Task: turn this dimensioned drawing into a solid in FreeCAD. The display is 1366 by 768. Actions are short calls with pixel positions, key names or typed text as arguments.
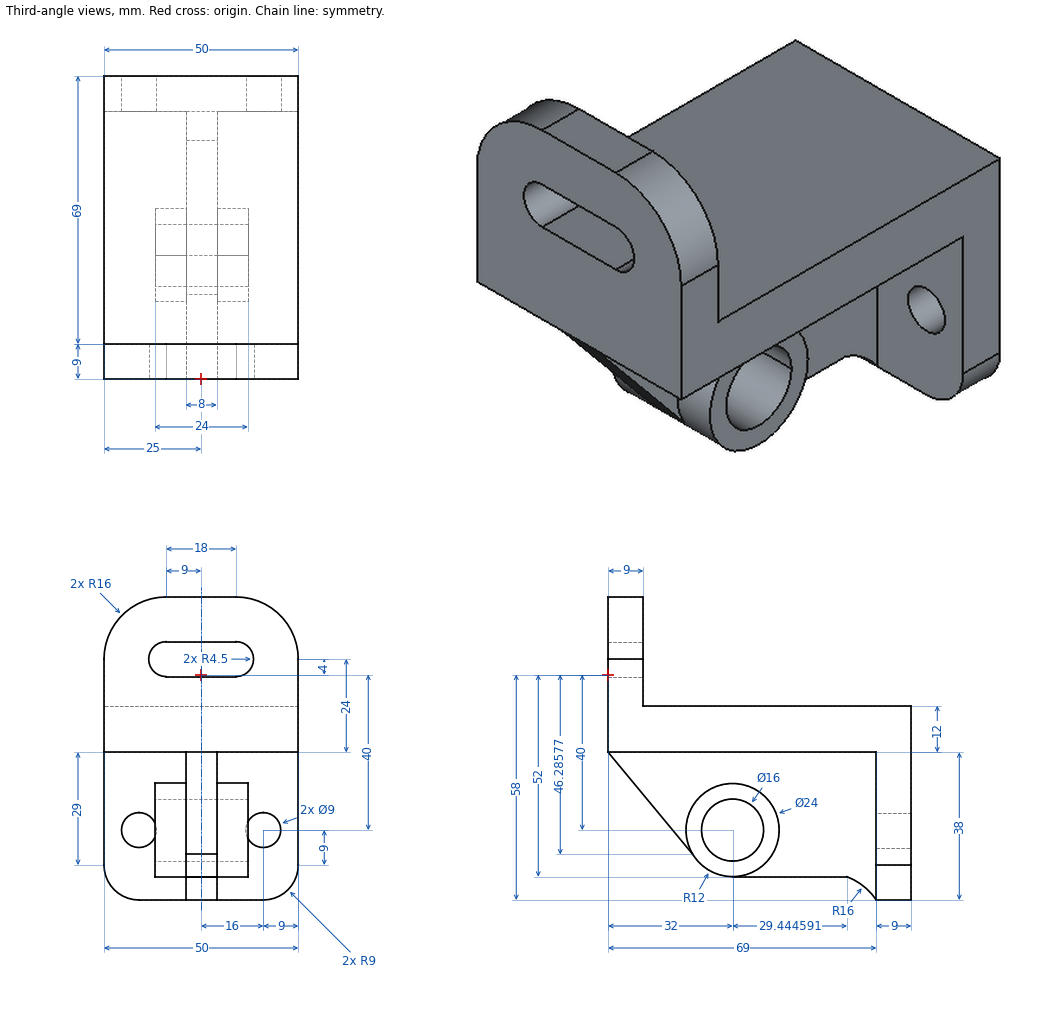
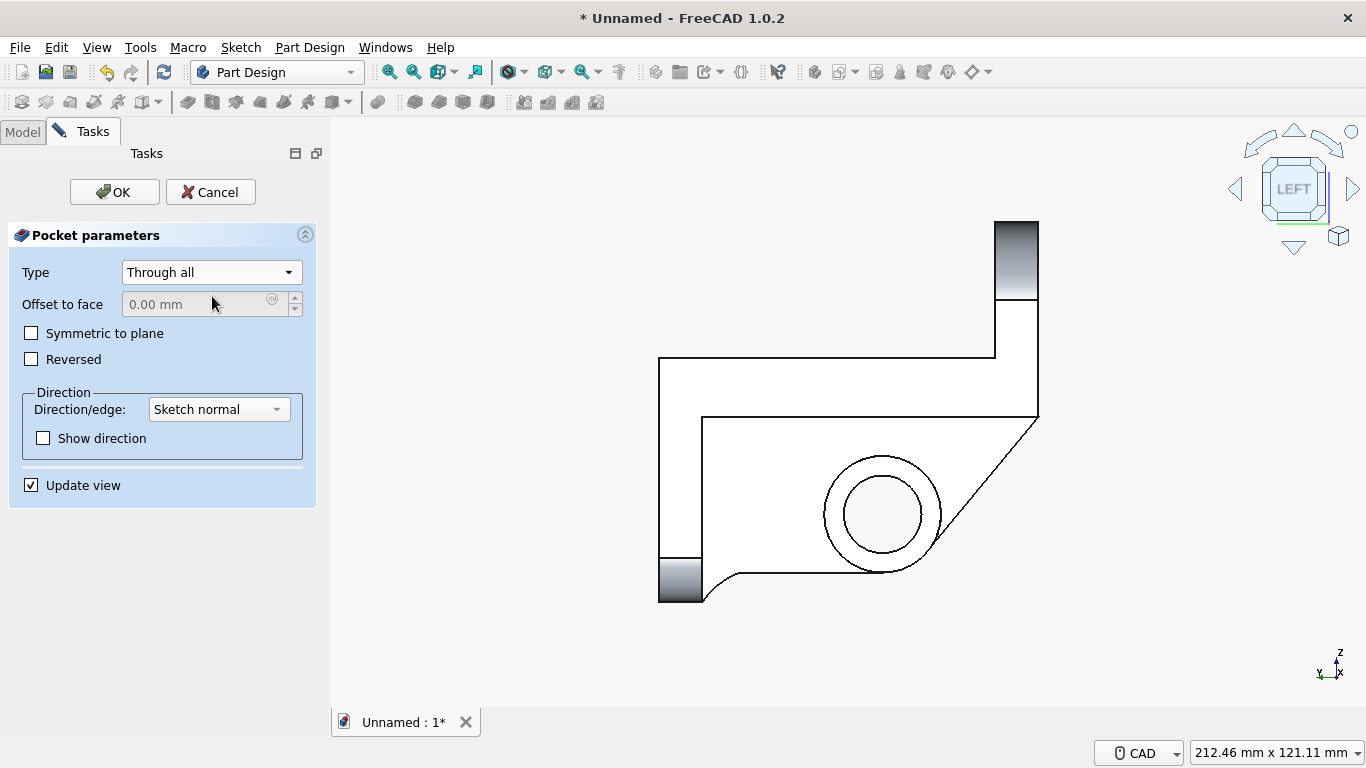
click(115, 192)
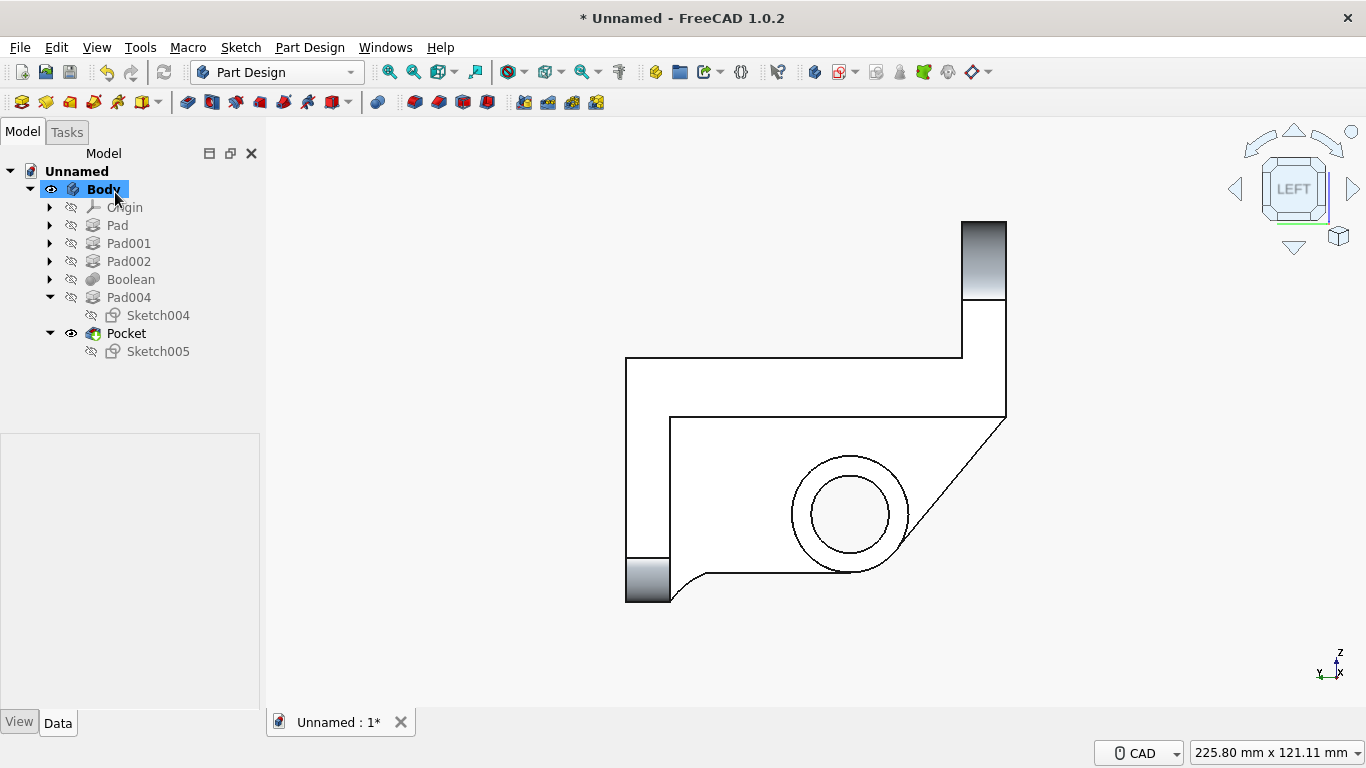
key(0)